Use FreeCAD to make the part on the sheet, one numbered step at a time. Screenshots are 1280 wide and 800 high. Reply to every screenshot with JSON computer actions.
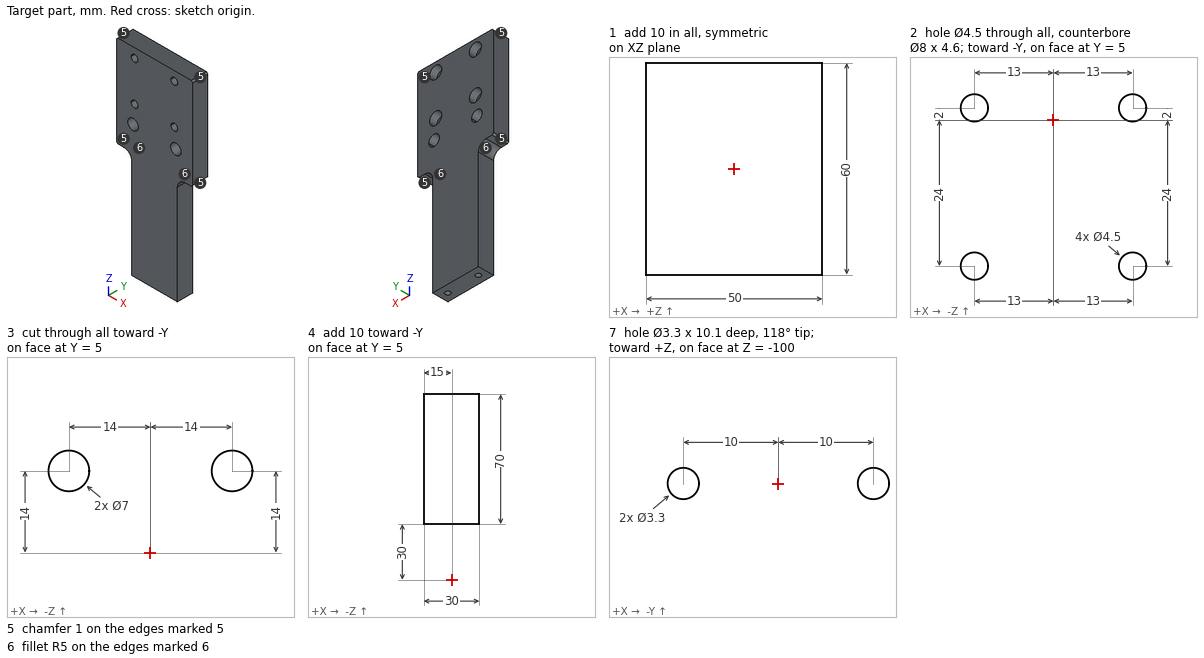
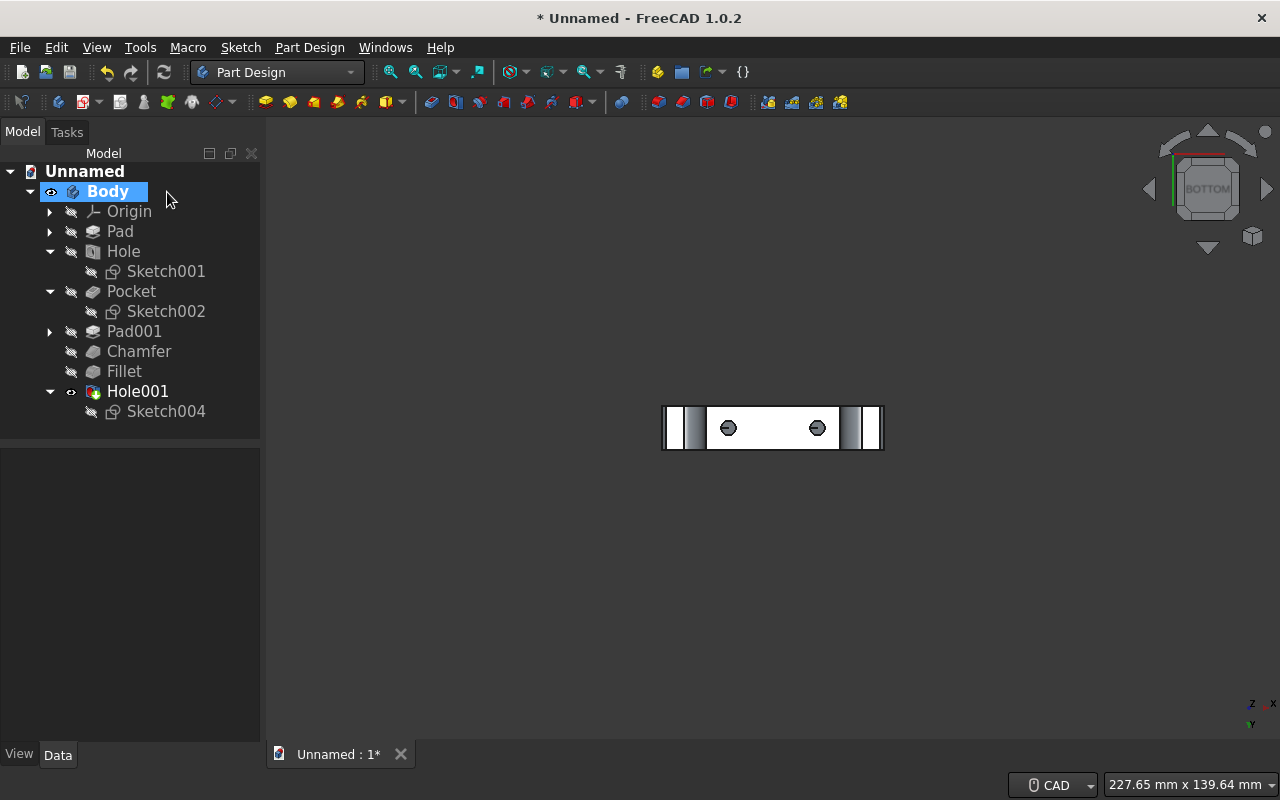
{"action": "key", "text": "0"}